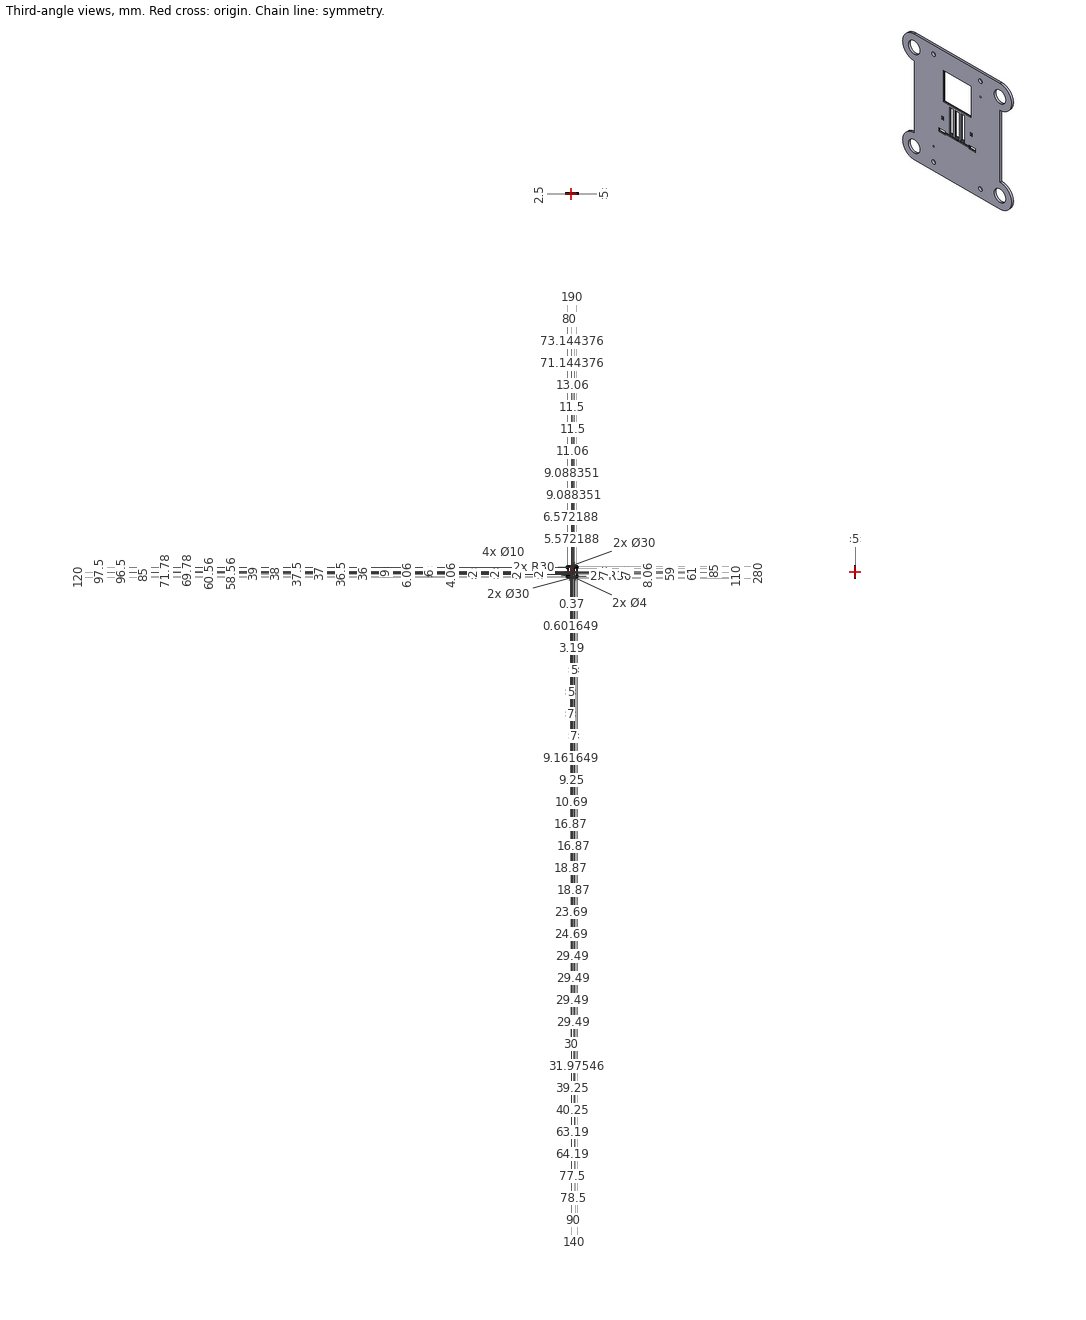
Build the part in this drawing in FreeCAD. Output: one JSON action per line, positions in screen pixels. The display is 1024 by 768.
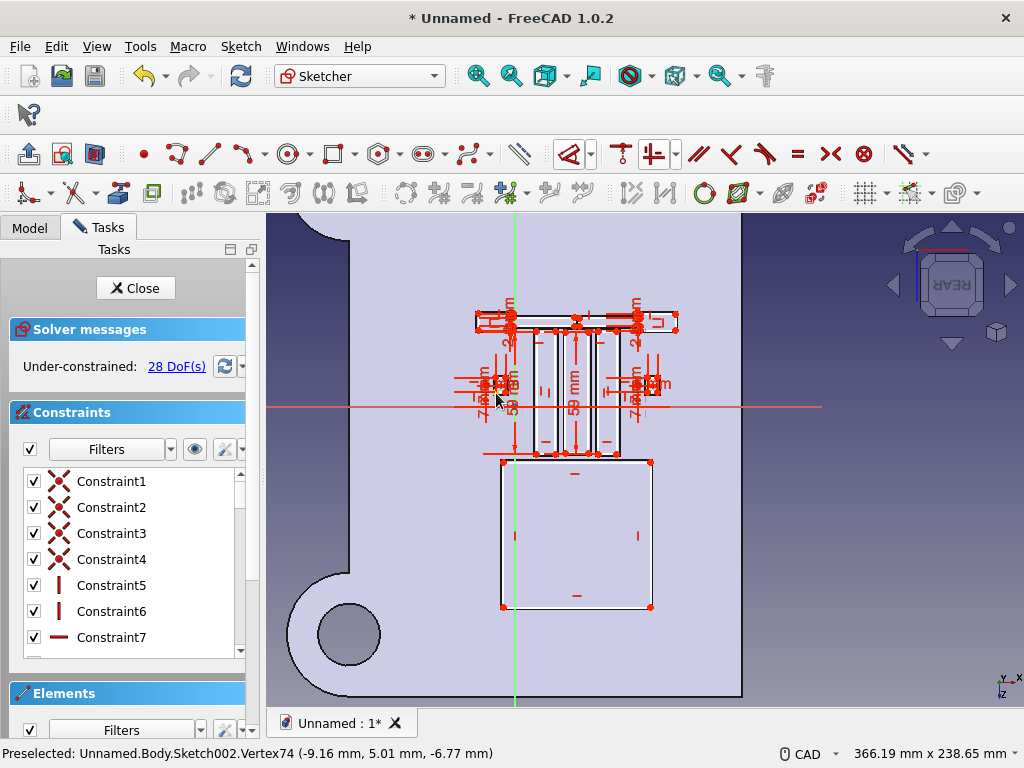
{"action": "scroll", "coordinate": [513, 331], "scroll_direction": "up", "scroll_amount": 6}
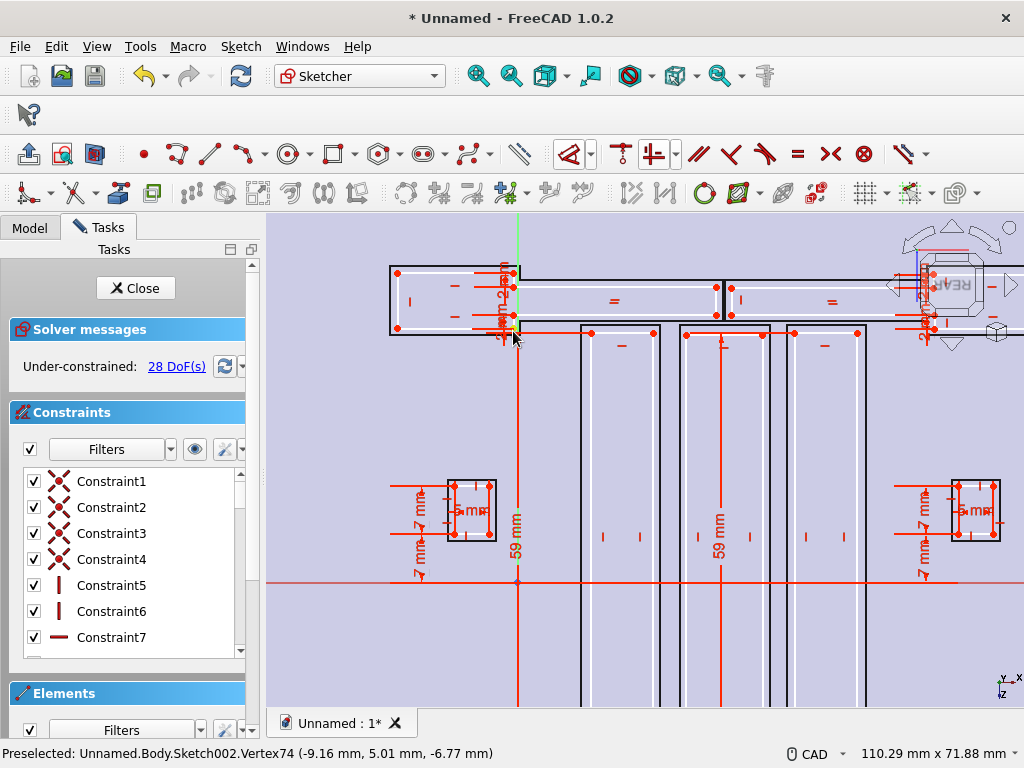
{"action": "left_click", "coordinate": [514, 329]}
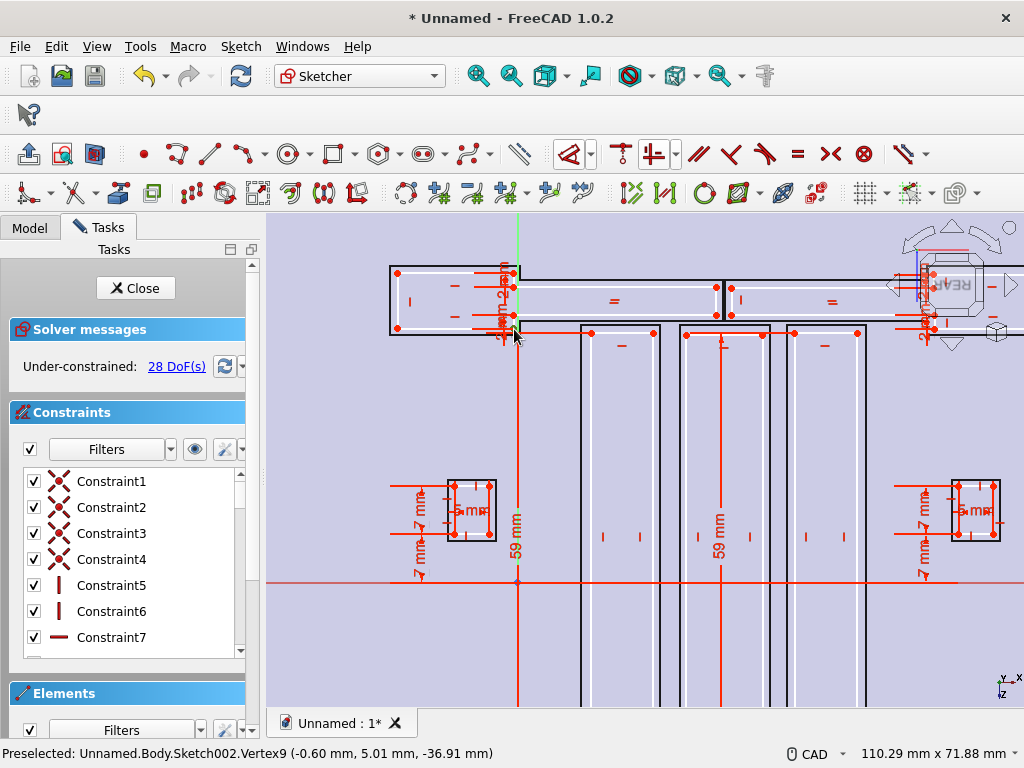
{"action": "left_click", "coordinate": [590, 154]}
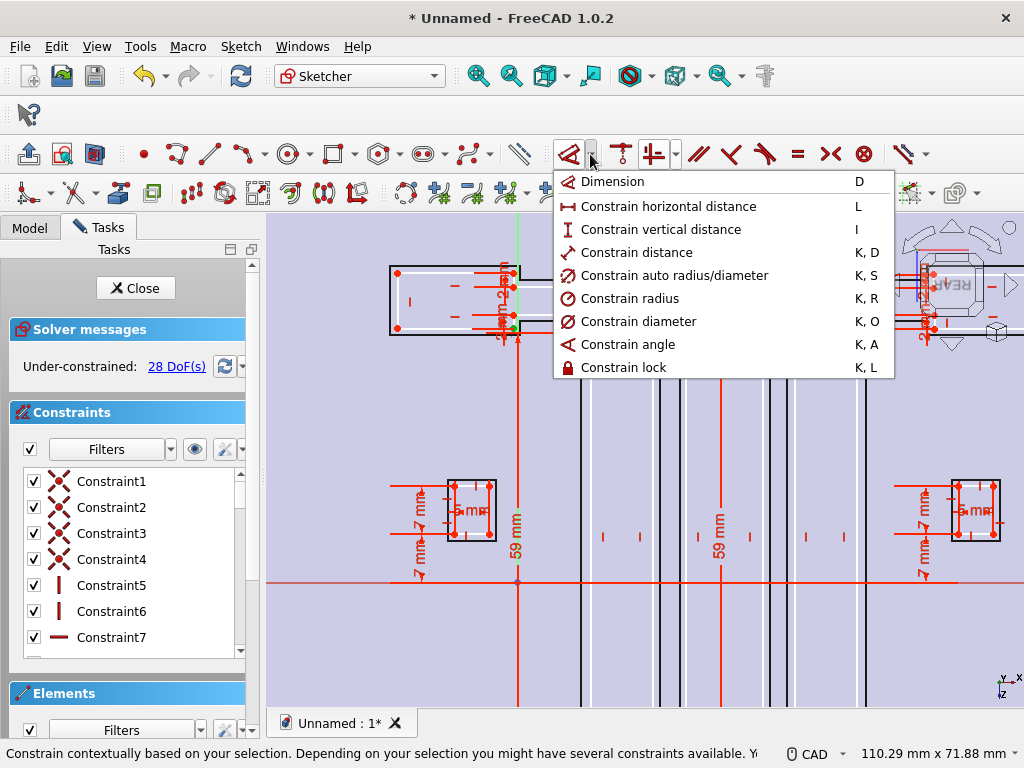
{"action": "left_click", "coordinate": [724, 230]}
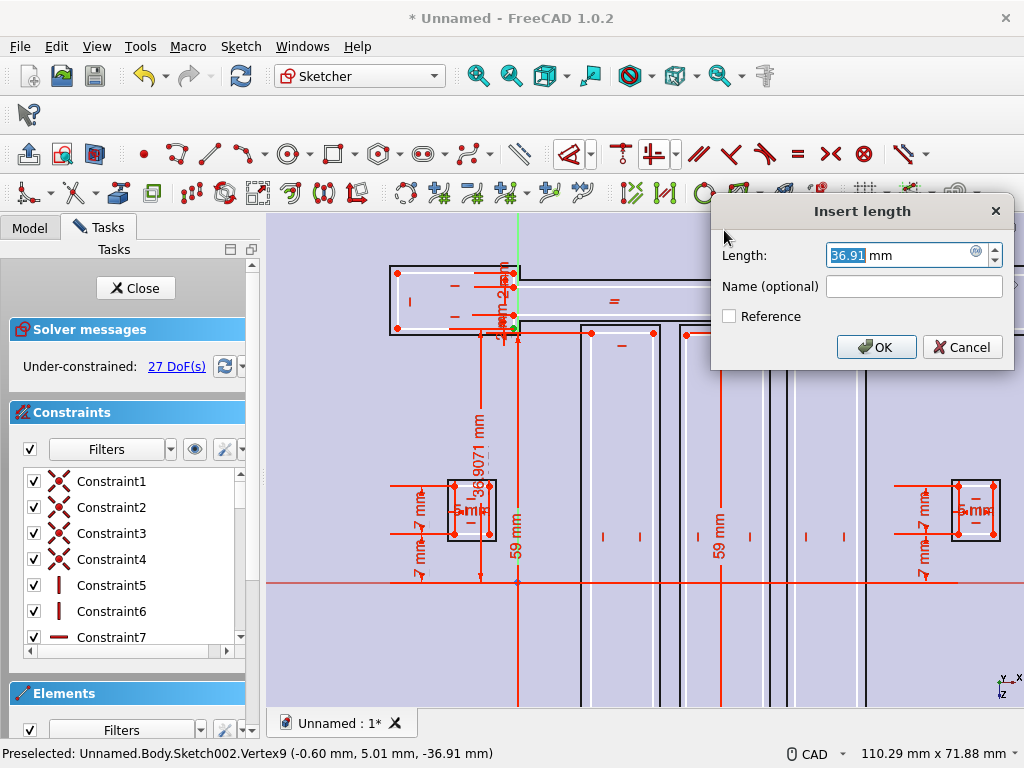
{"action": "type", "text": "37"}
{"action": "key", "text": "Return"}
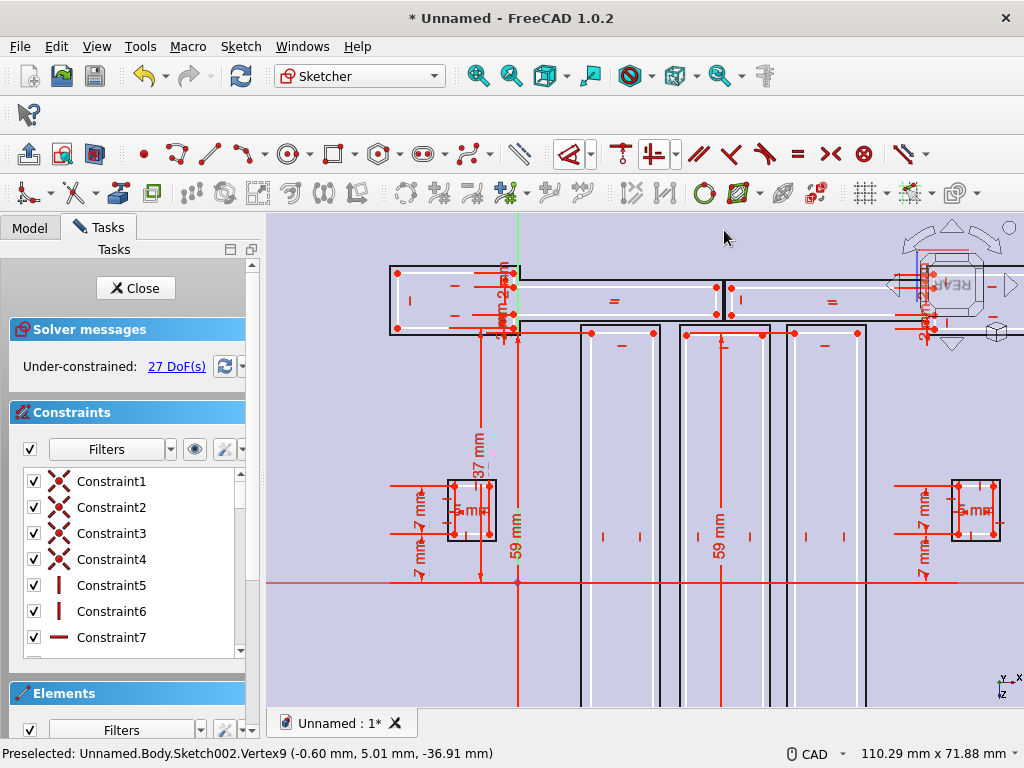
{"action": "left_click", "coordinate": [732, 315]}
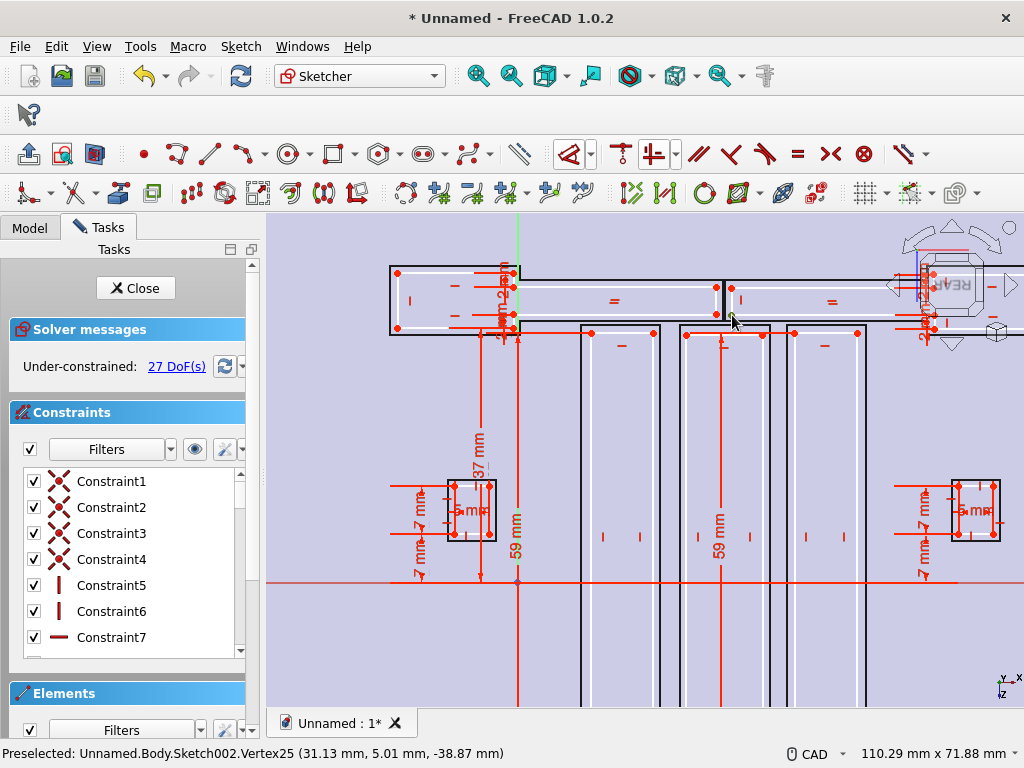
{"action": "left_click", "coordinate": [590, 154]}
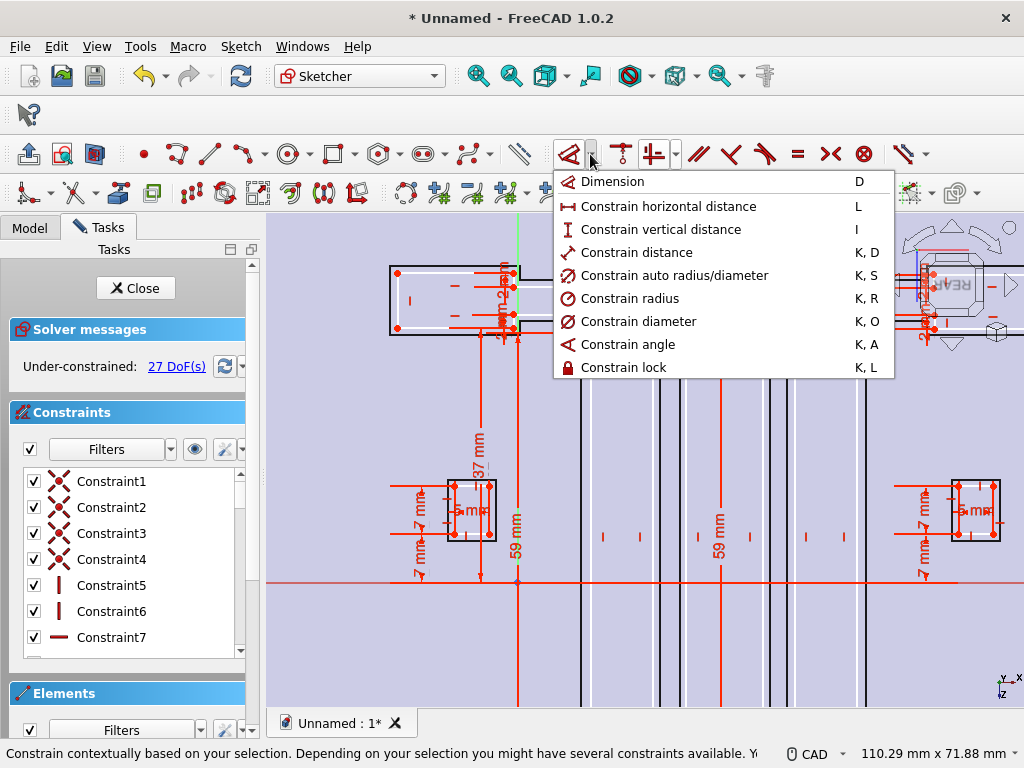
{"action": "left_click", "coordinate": [724, 230]}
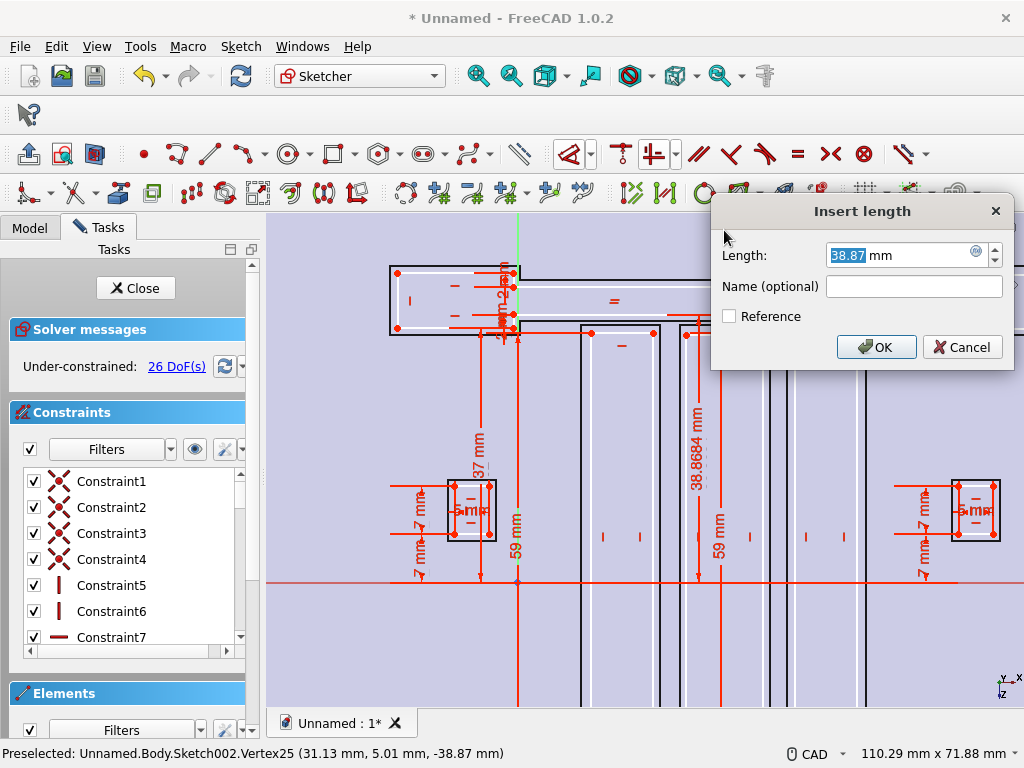
{"action": "type", "text": "39"}
{"action": "key", "text": "Return"}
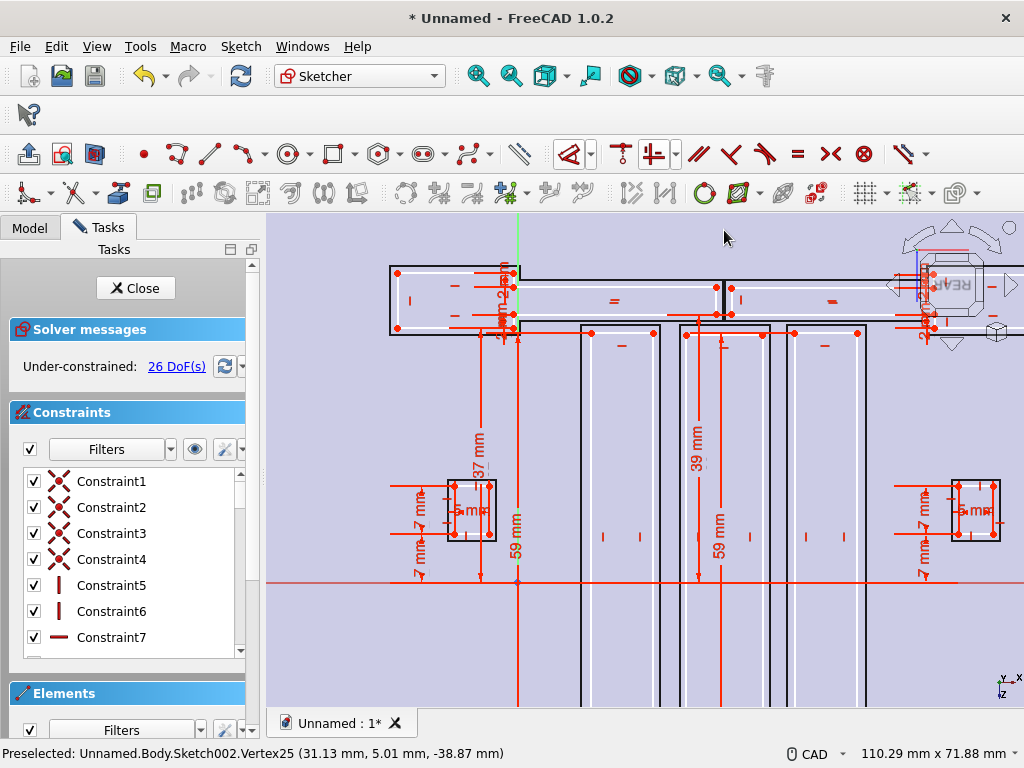
{"action": "scroll", "coordinate": [716, 304], "scroll_direction": "up", "scroll_amount": 2}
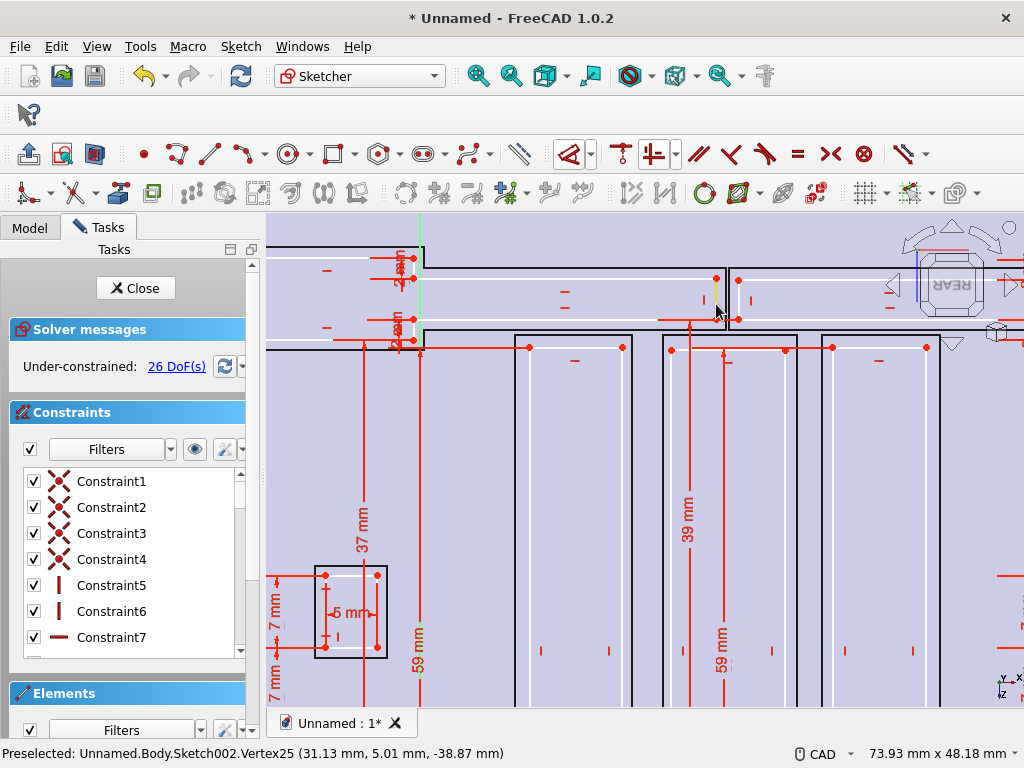
{"action": "left_click", "coordinate": [716, 303]}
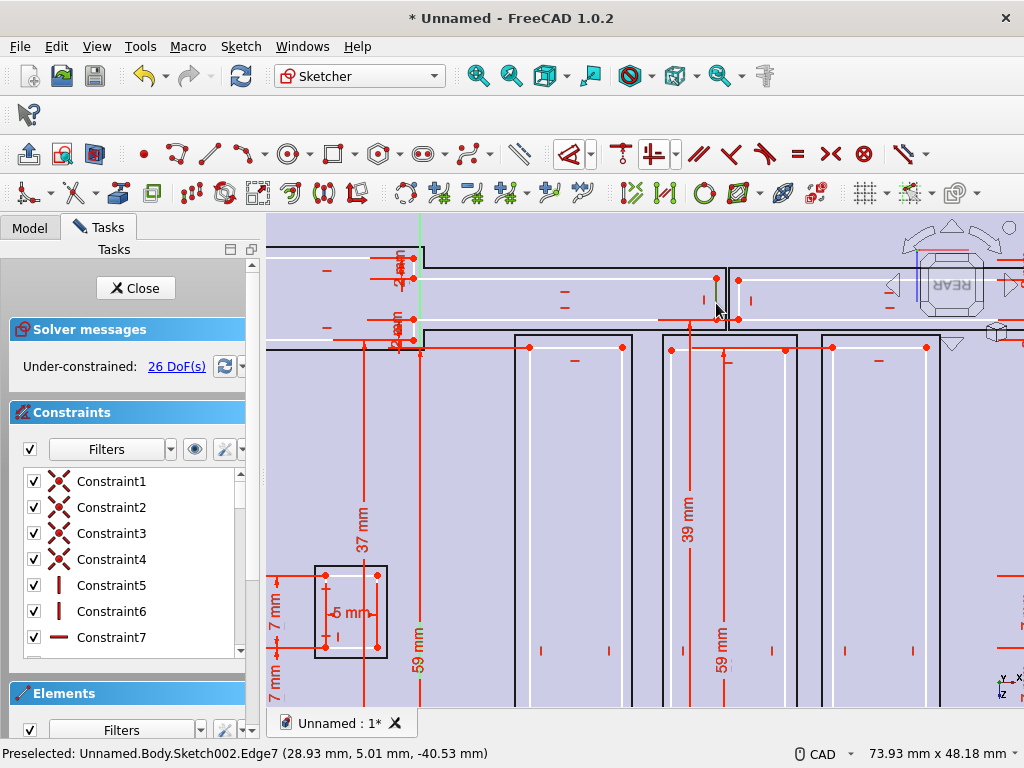
{"action": "left_click", "coordinate": [590, 154]}